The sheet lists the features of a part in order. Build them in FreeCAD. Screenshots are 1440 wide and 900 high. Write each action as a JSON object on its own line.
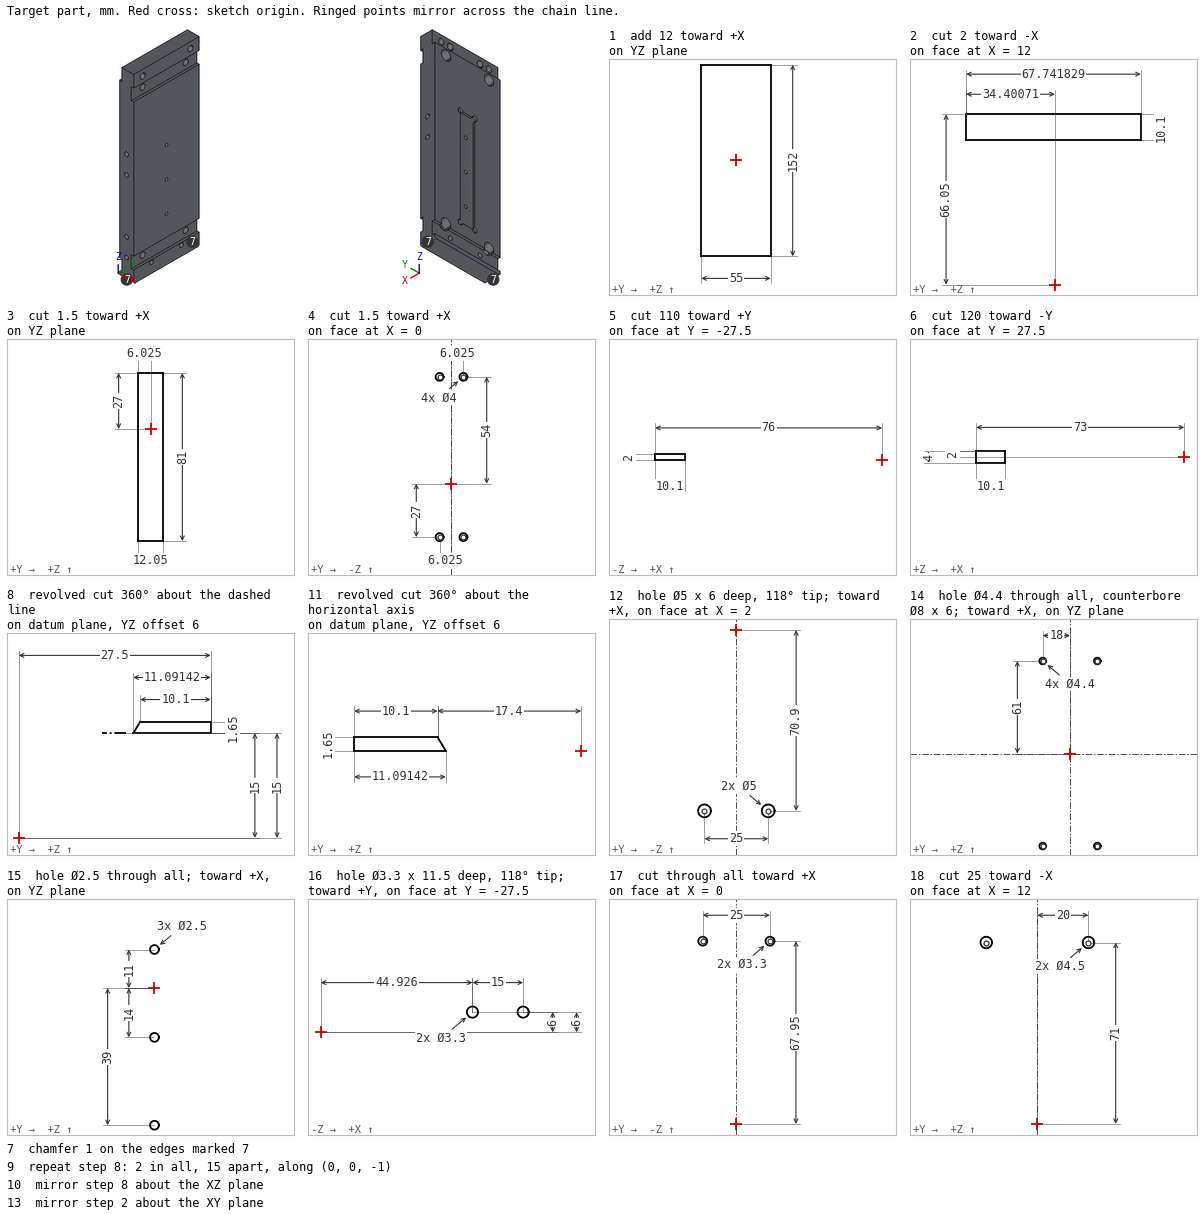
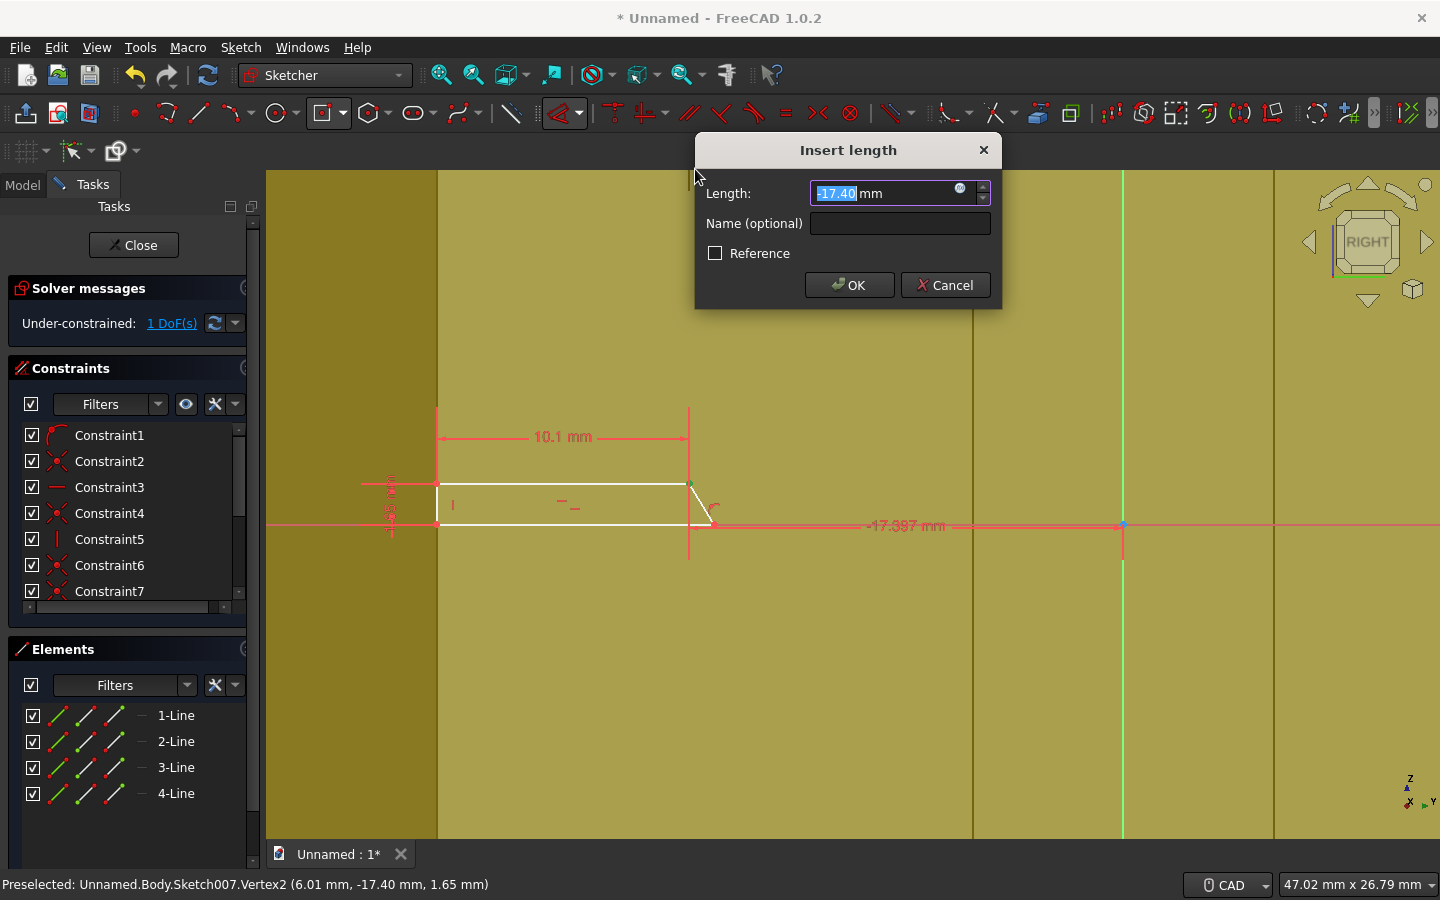
{"action": "type", "text": "-17.4"}
{"action": "key", "text": "Return"}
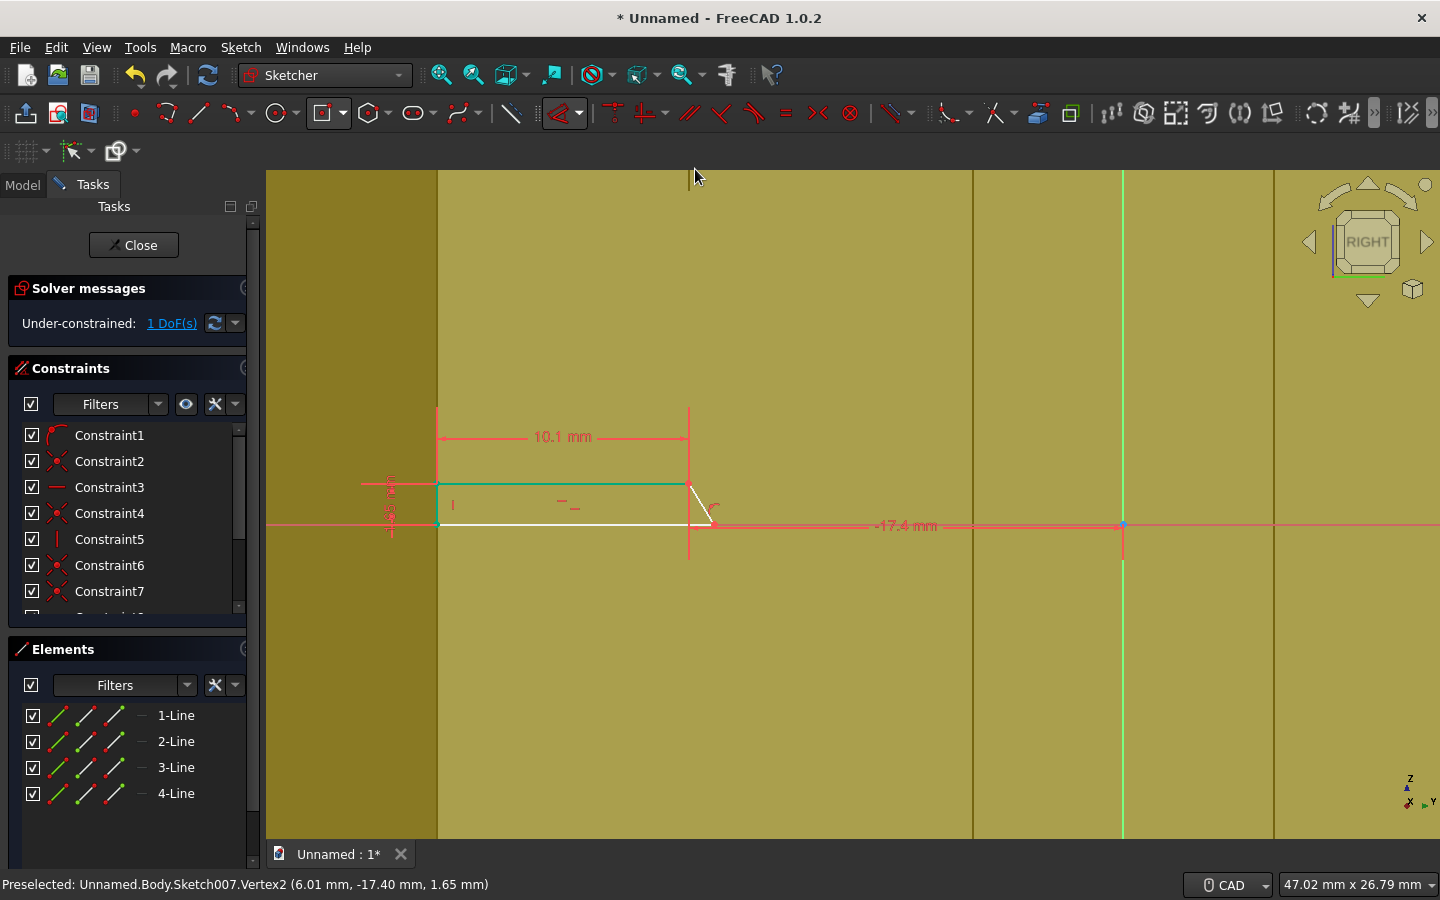
{"action": "left_click", "coordinate": [520, 525]}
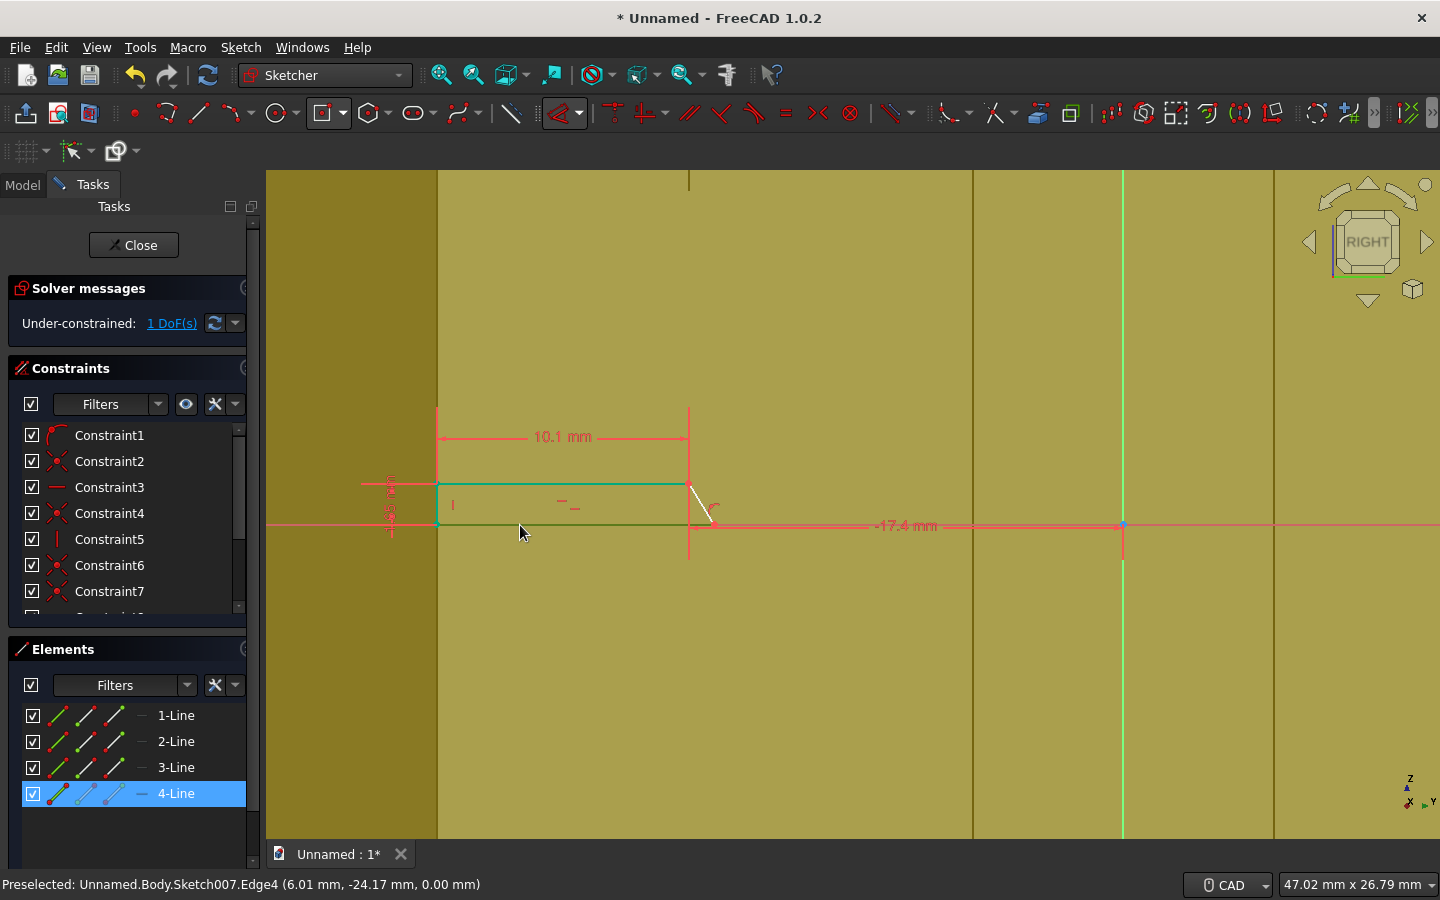
{"action": "key", "text": "l"}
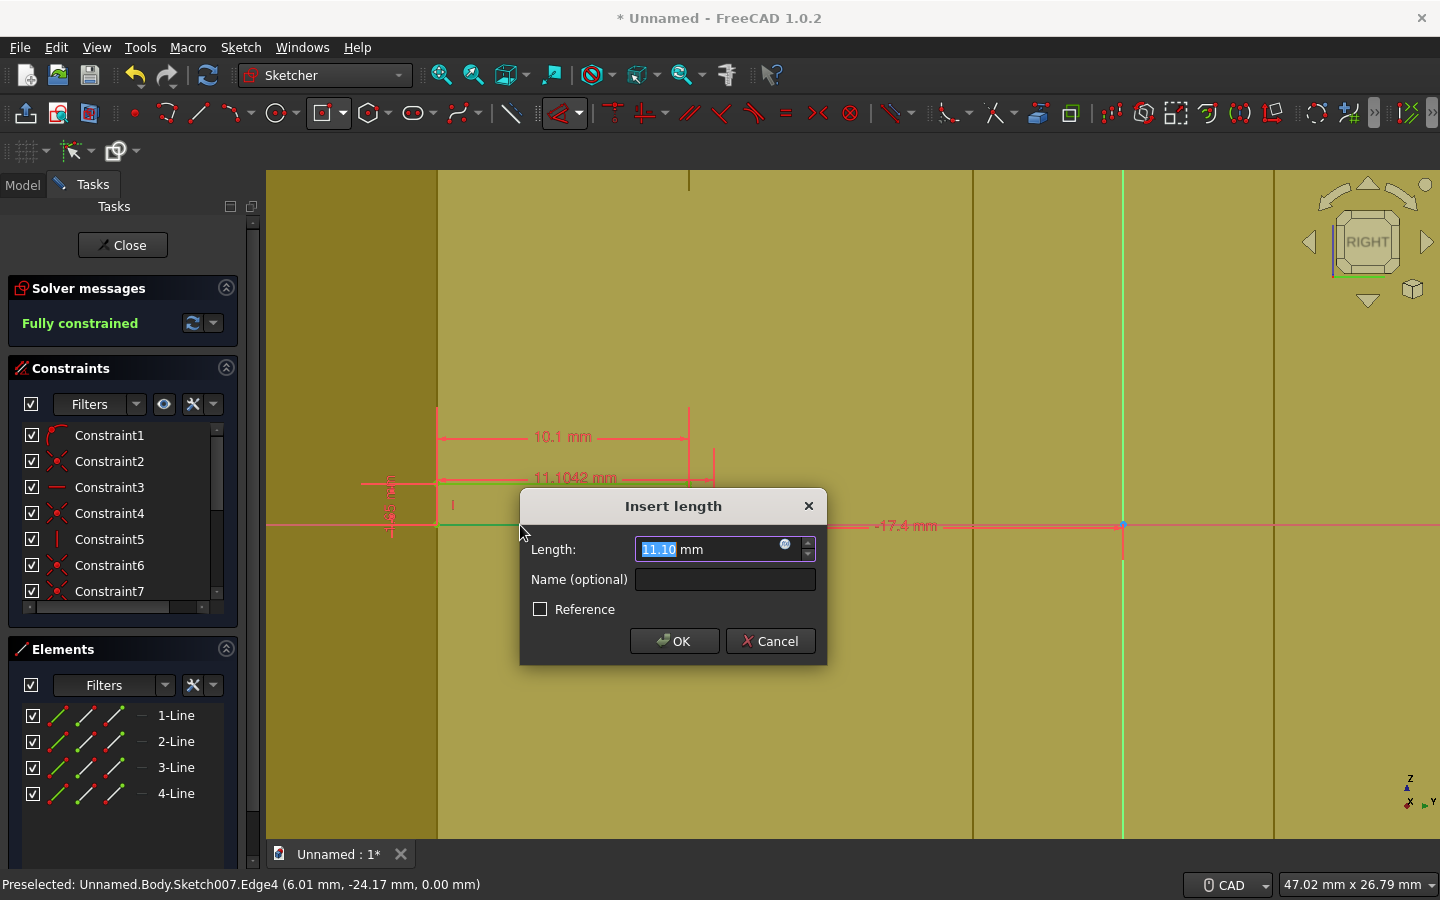
{"action": "type", "text": "11.09142"}
{"action": "key", "text": "Return"}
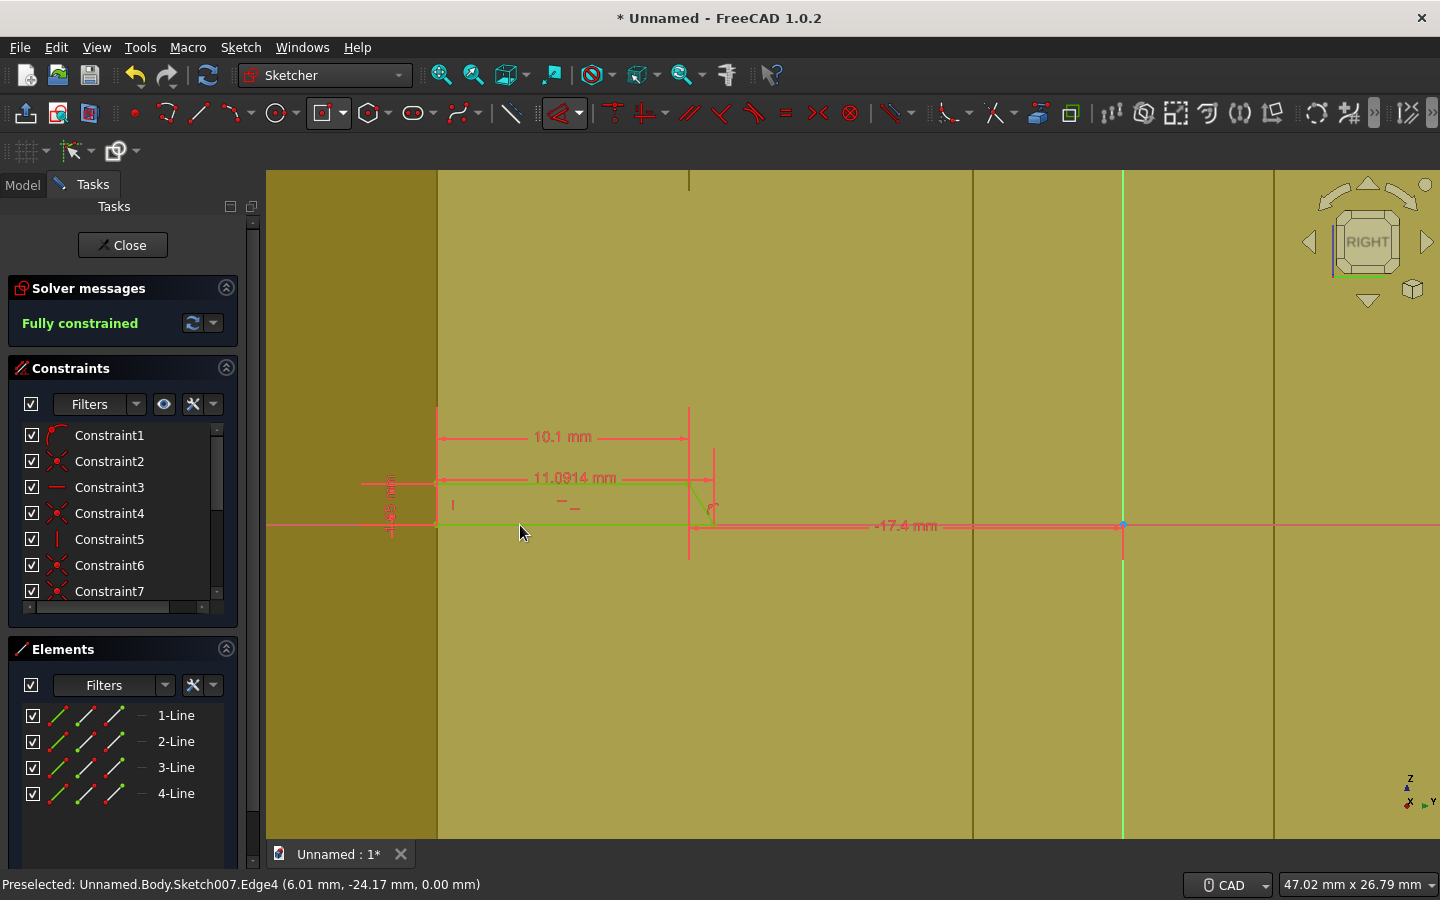
{"action": "left_click", "coordinate": [123, 245]}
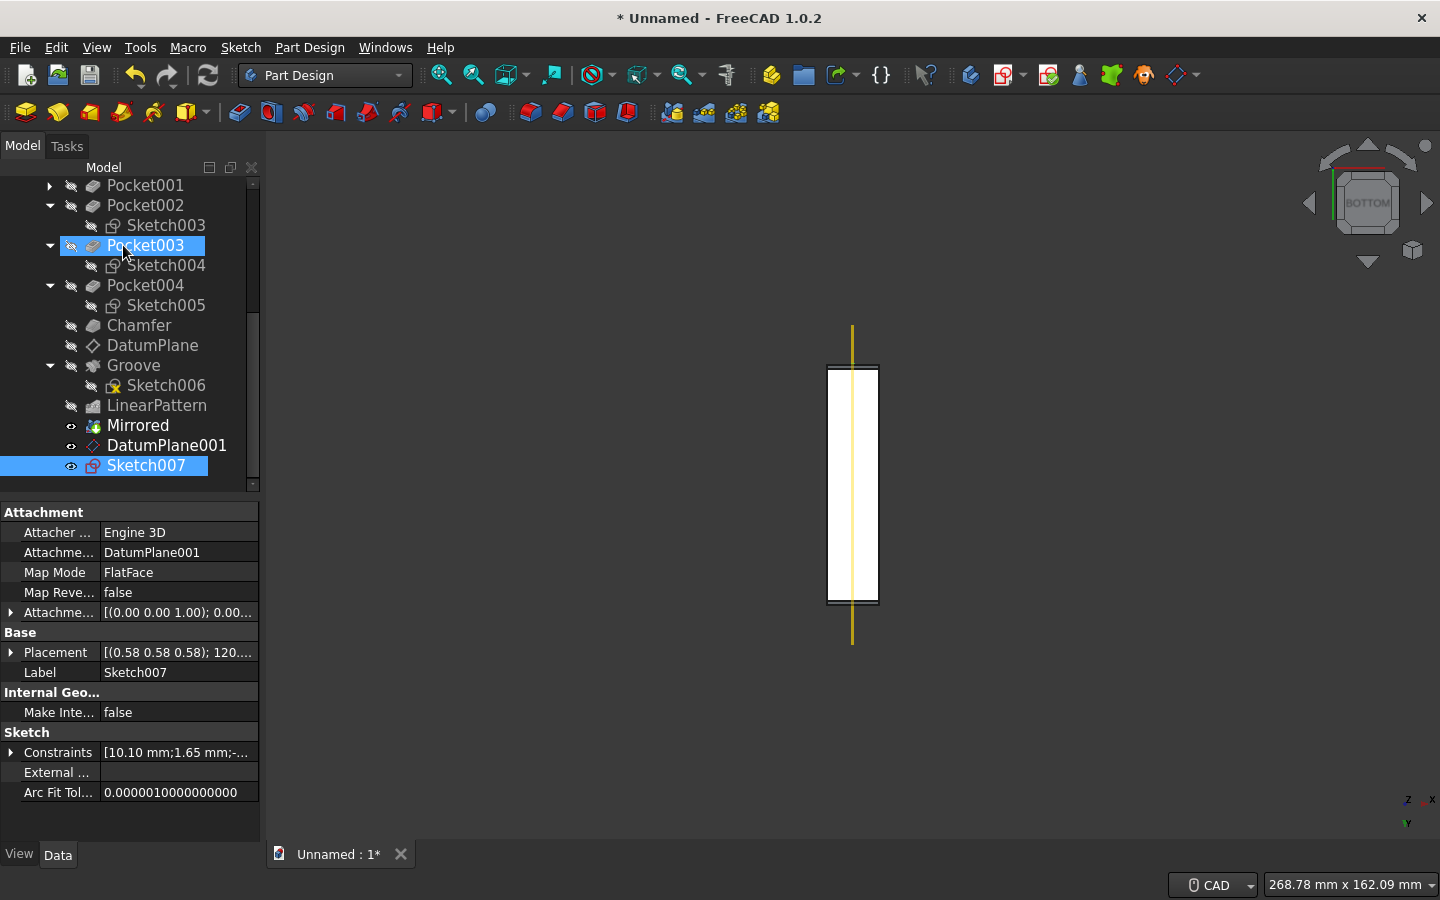
{"action": "left_click", "coordinate": [304, 112]}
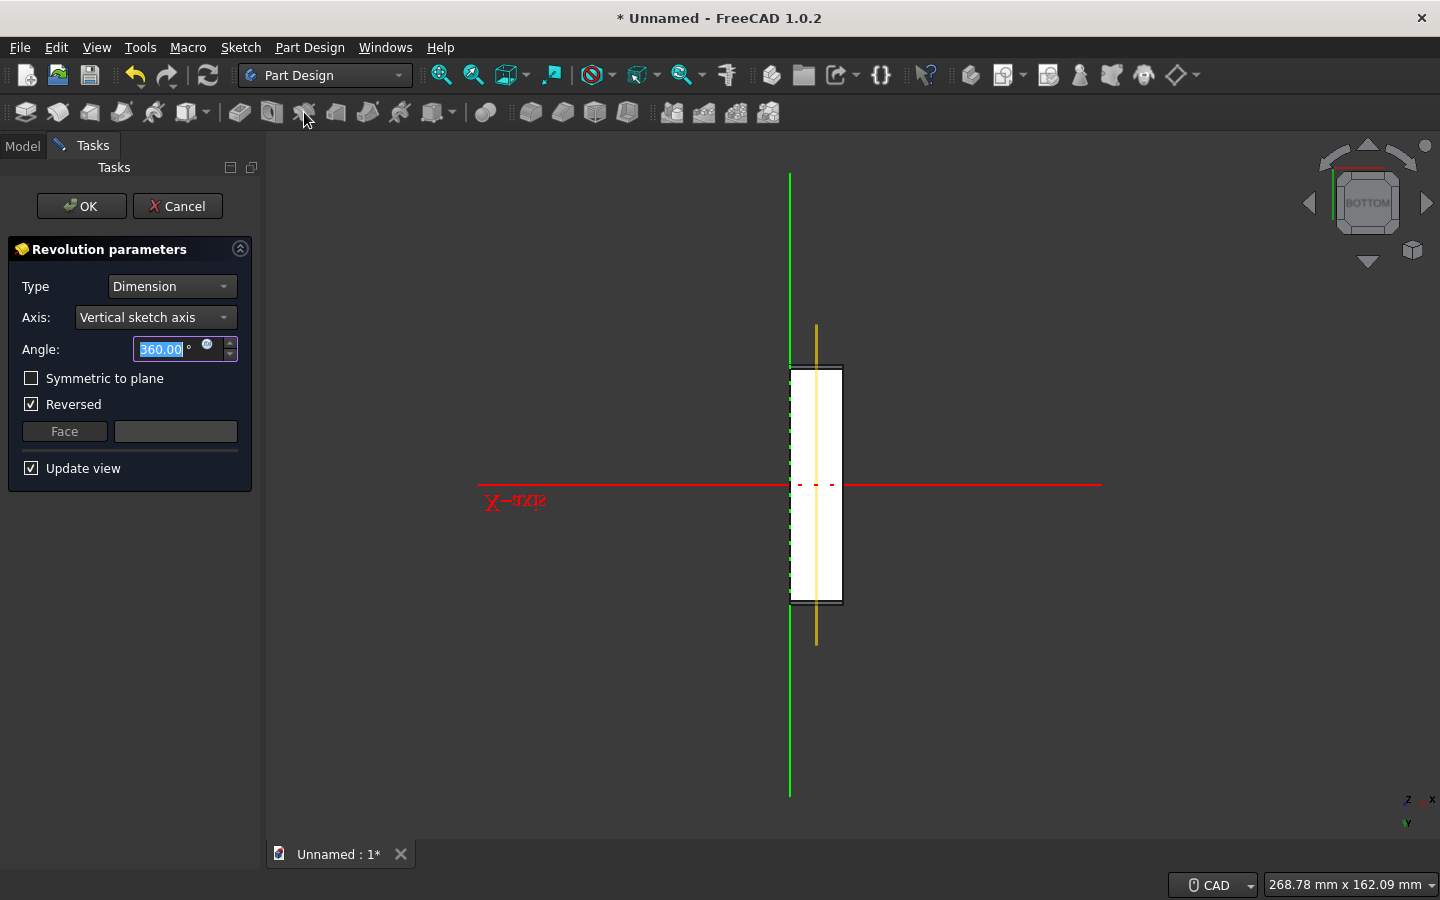
{"action": "left_click", "coordinate": [156, 318]}